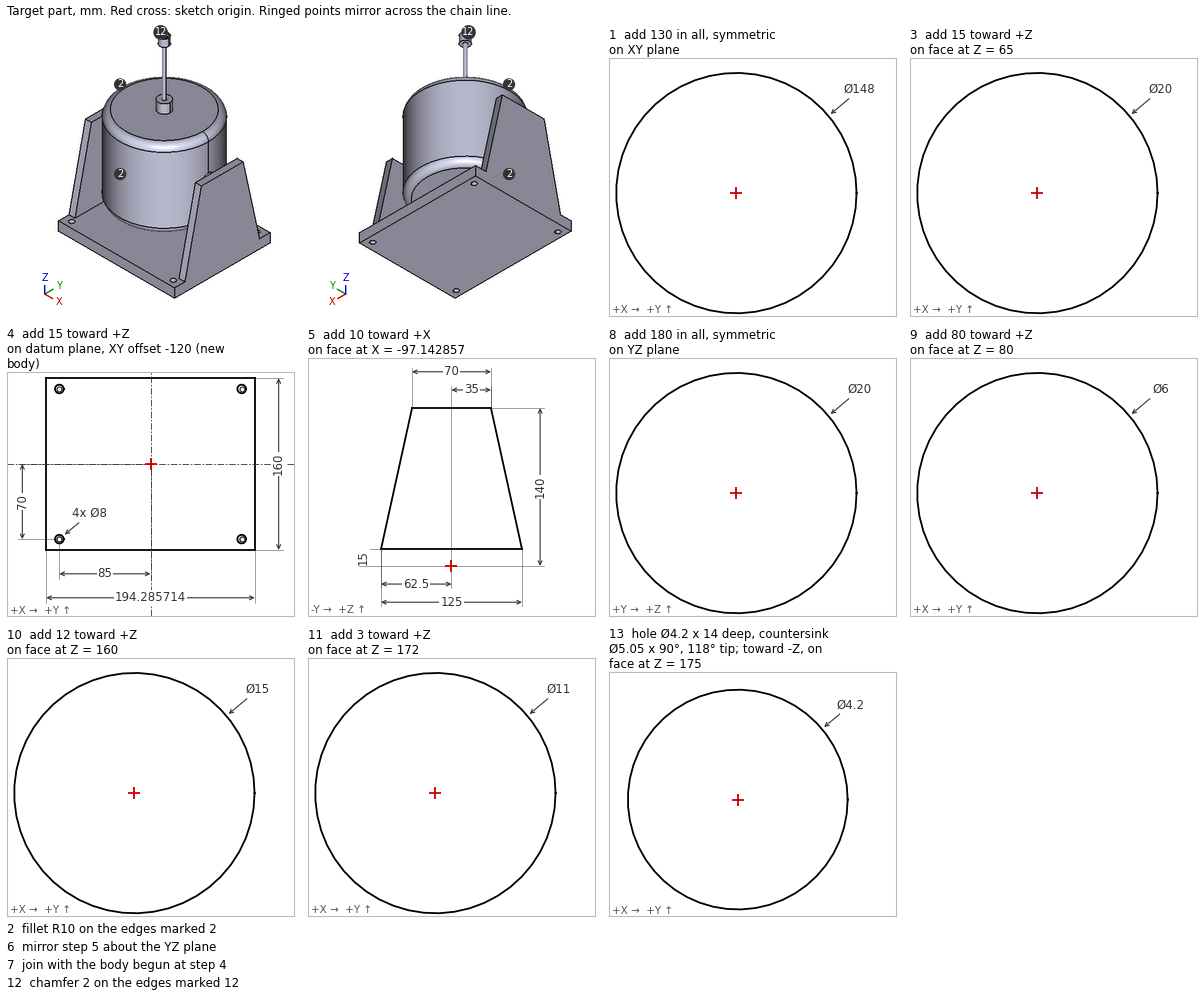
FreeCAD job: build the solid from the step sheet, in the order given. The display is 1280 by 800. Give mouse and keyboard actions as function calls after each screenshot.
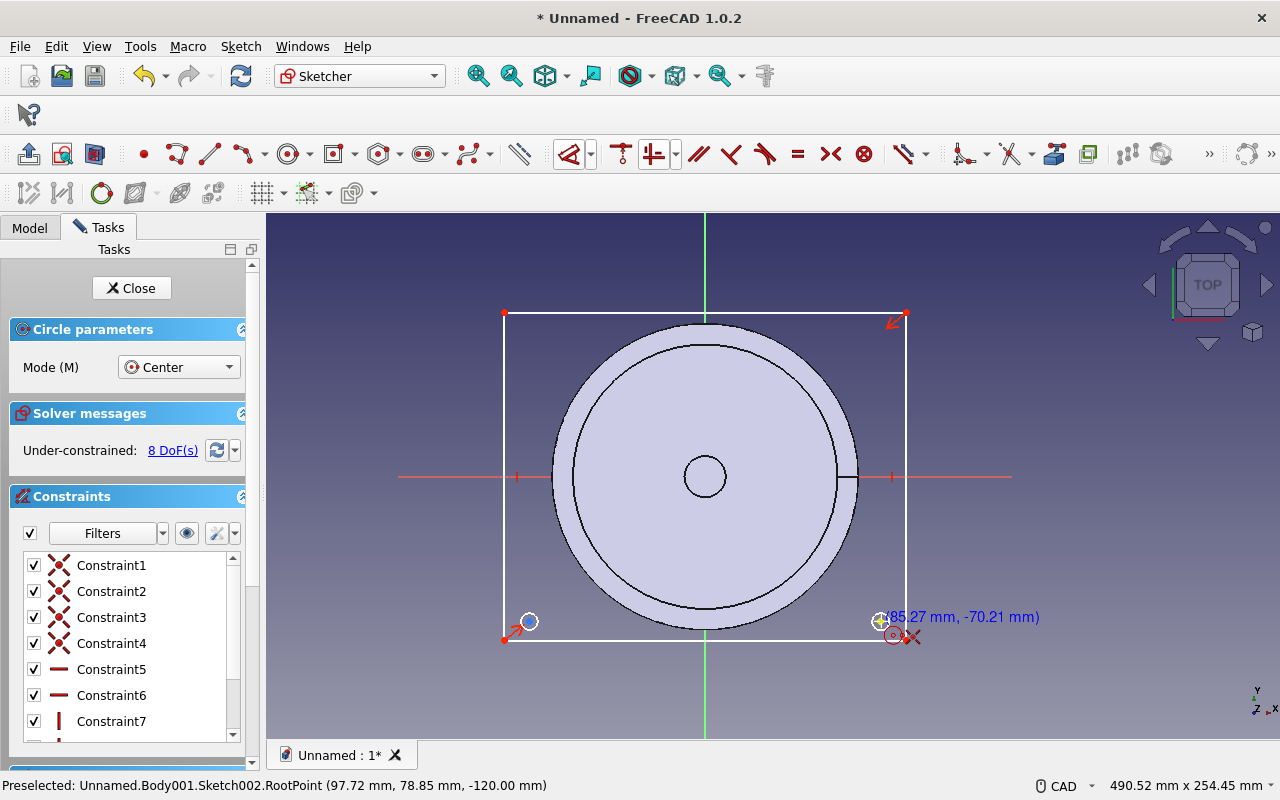
scroll(529, 332, up, 6)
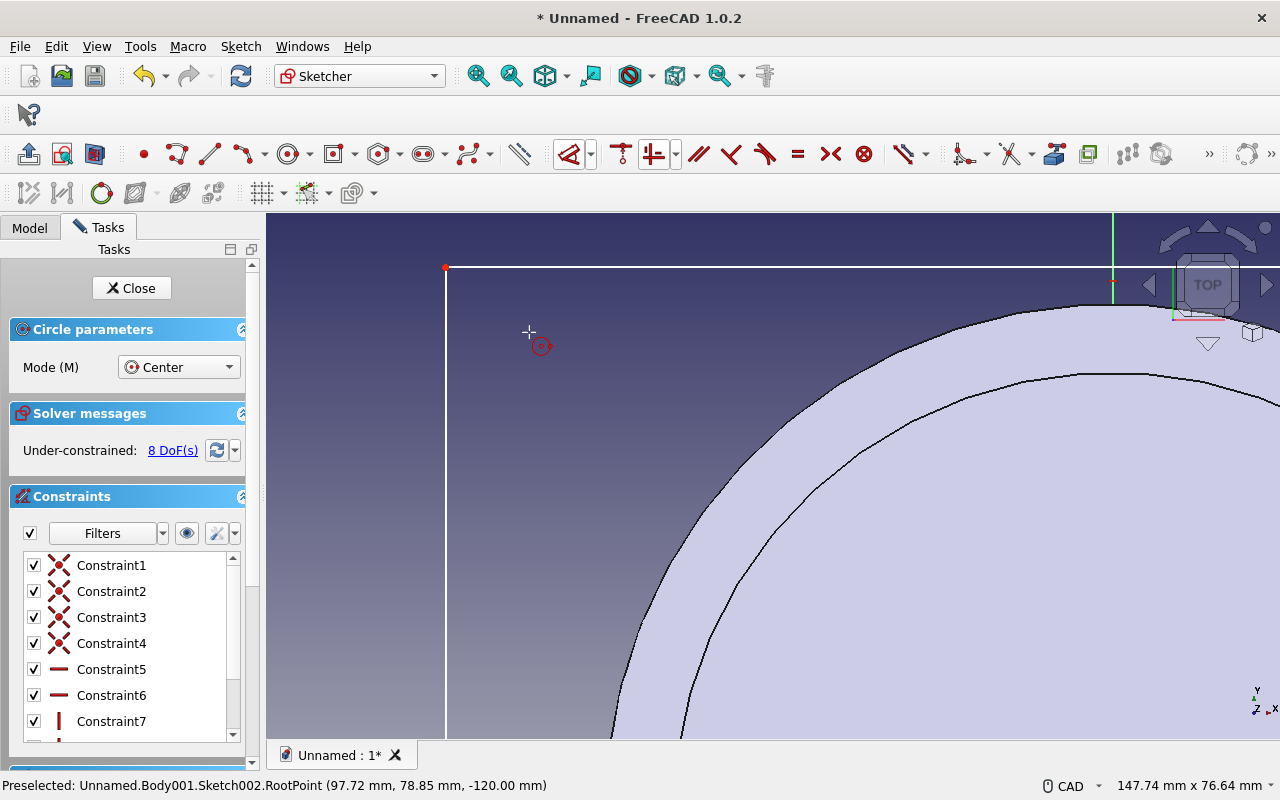
click(530, 331)
click(549, 312)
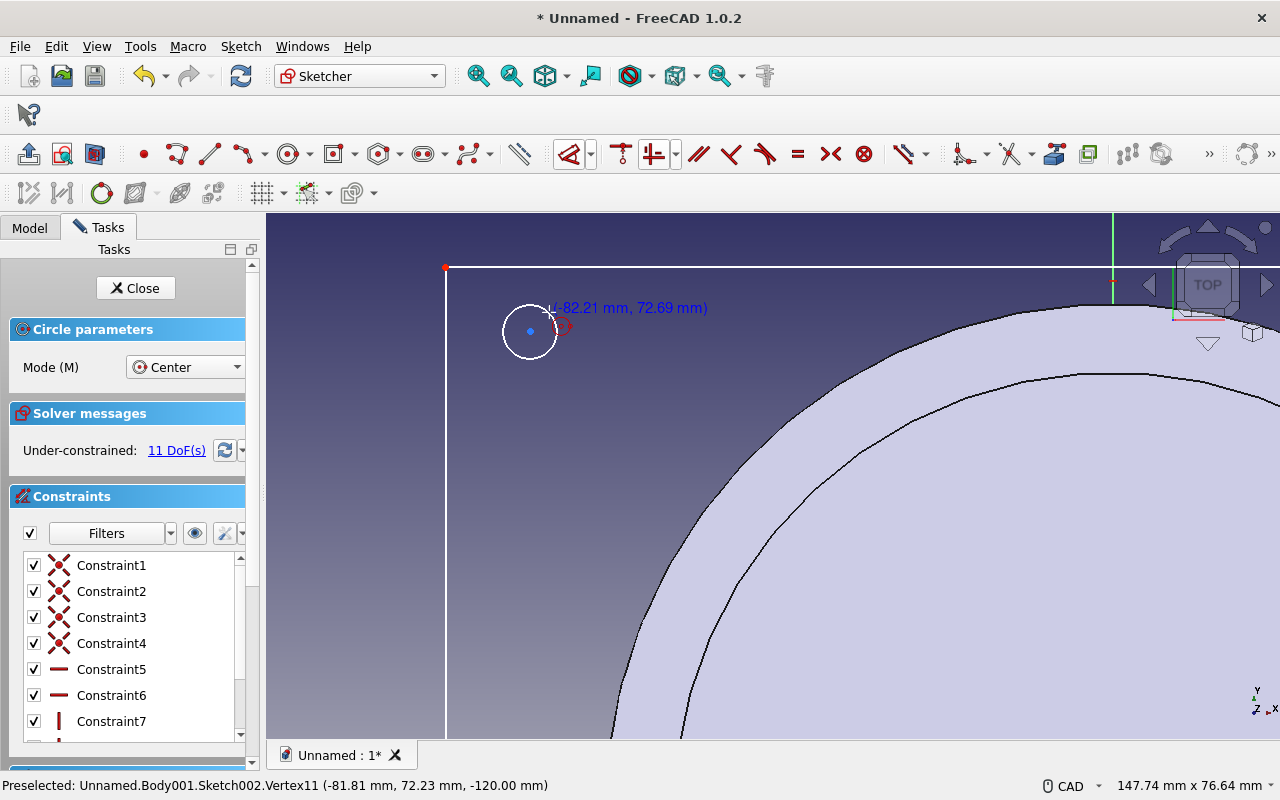
scroll(528, 331, down, 6)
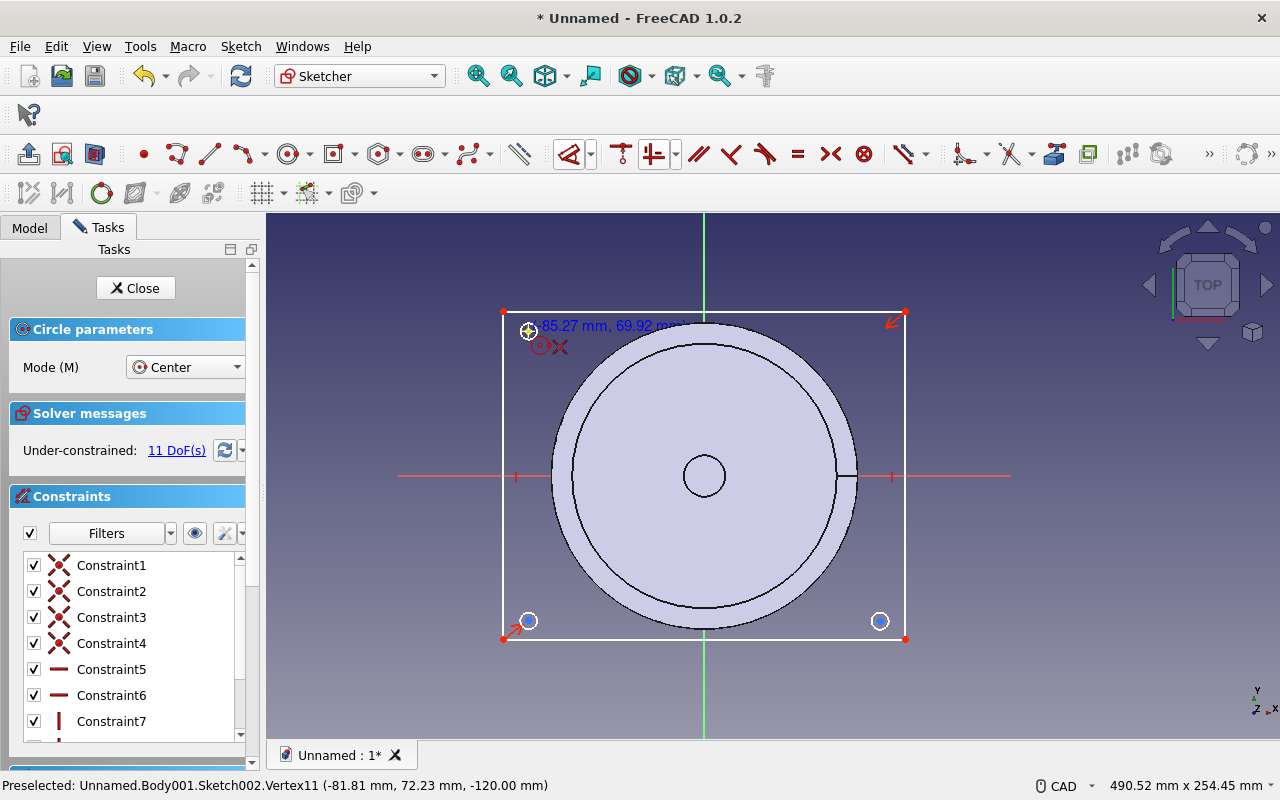
scroll(880, 331, up, 6)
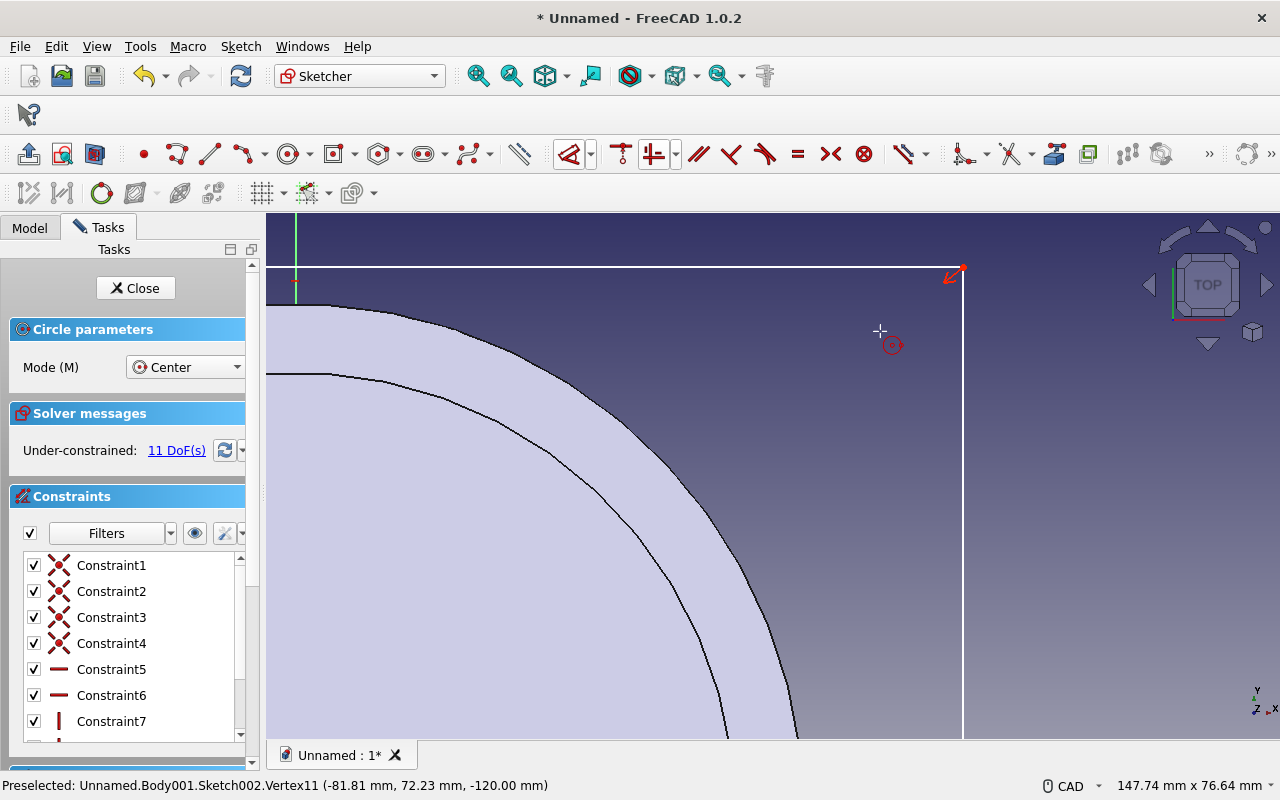
click(879, 331)
click(899, 312)
key(Escape)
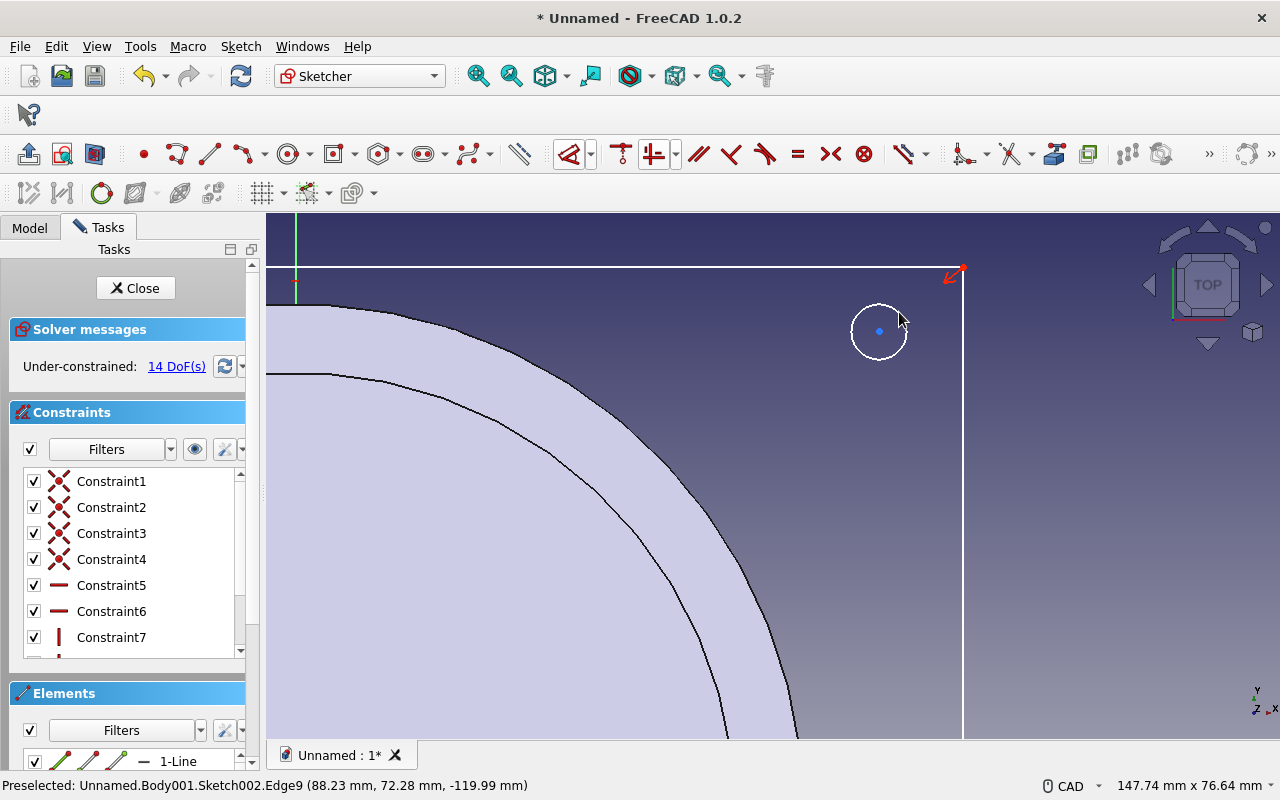
scroll(881, 331, down, 6)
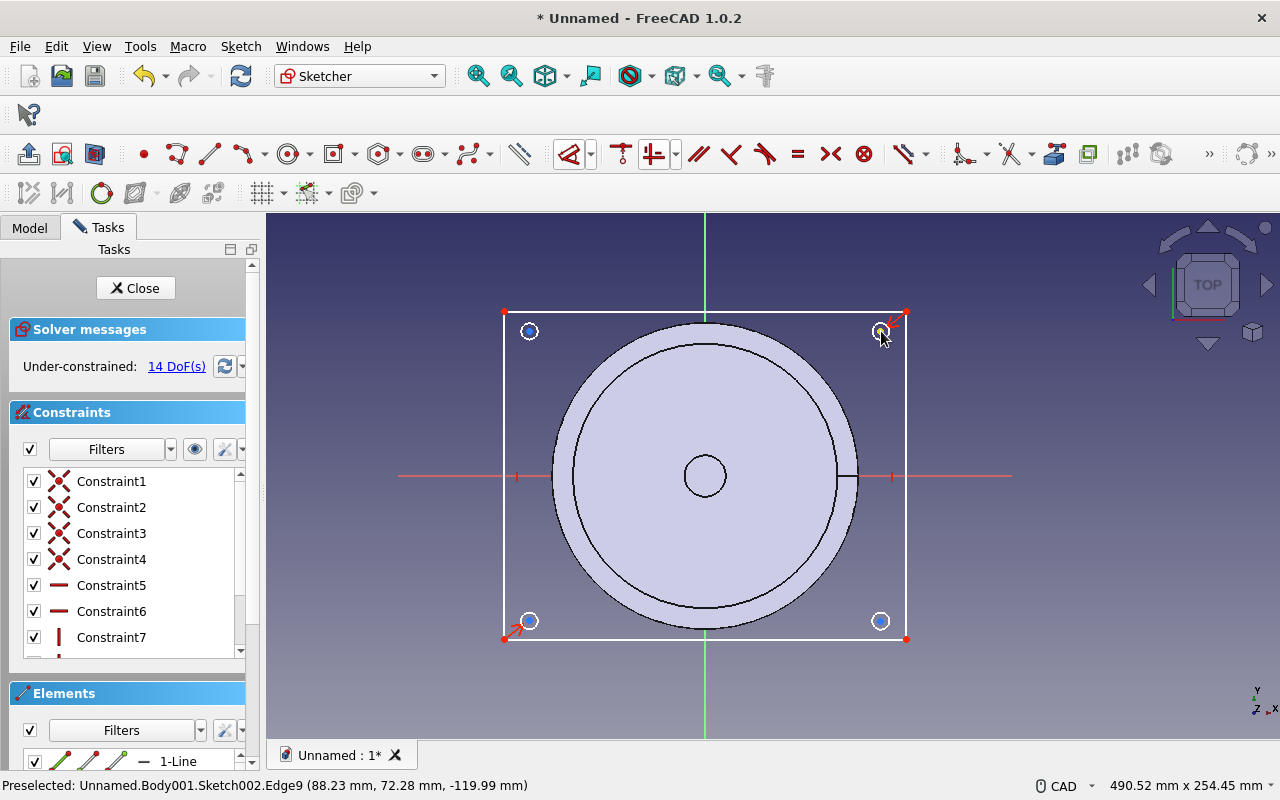
scroll(535, 615, up, 3)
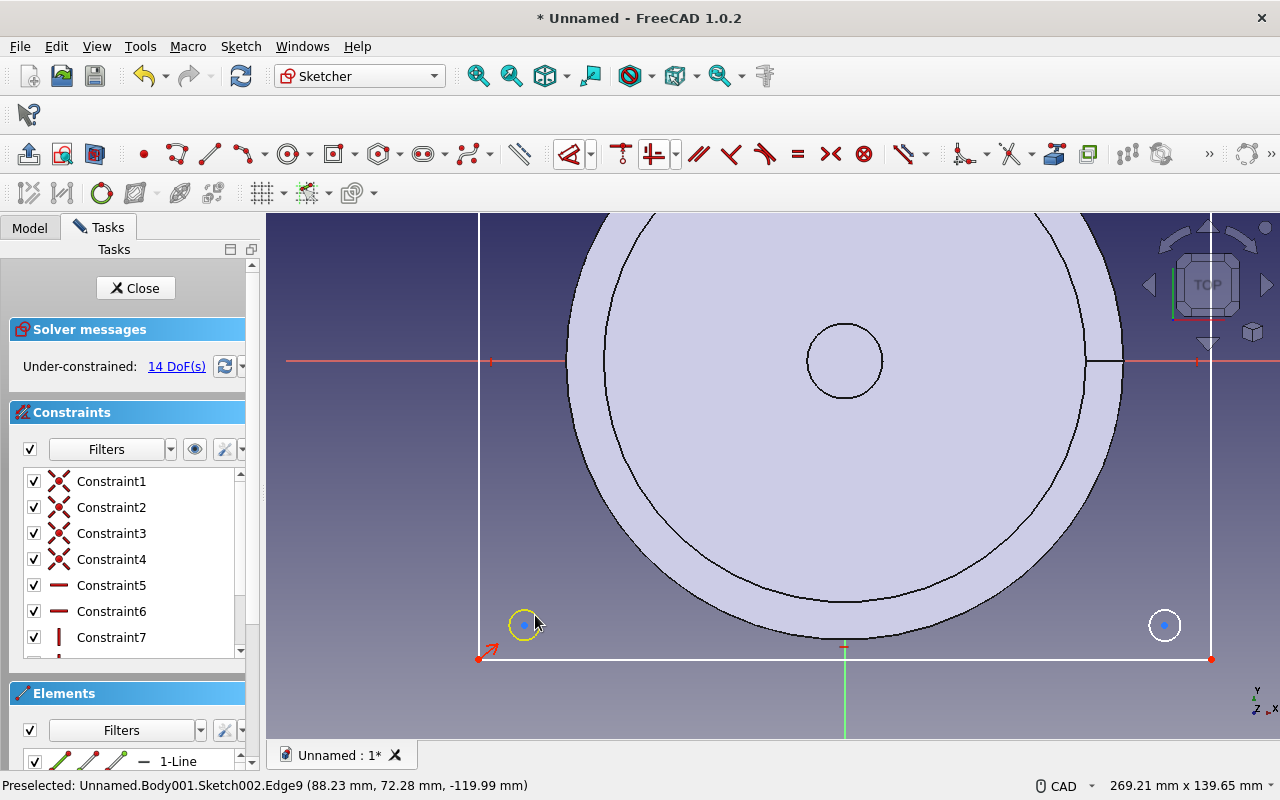
click(535, 614)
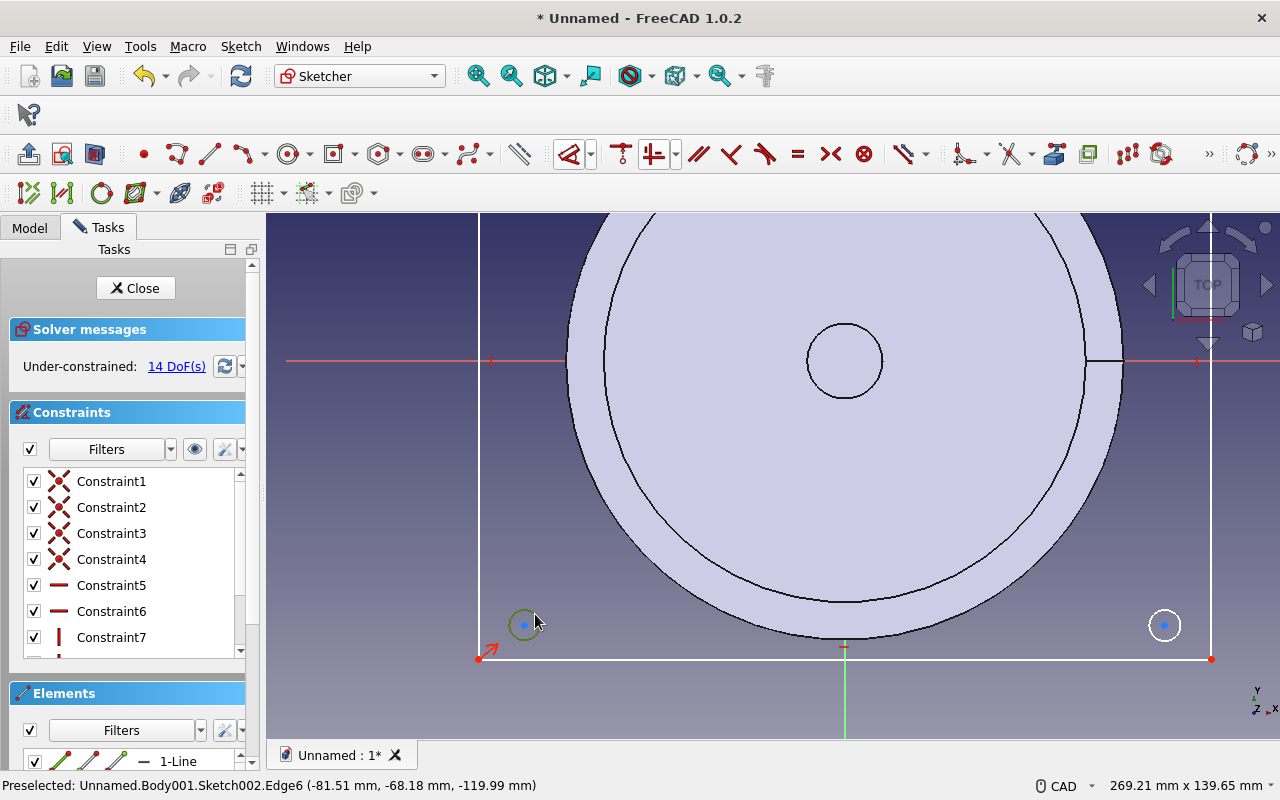
scroll(534, 616, down, 3)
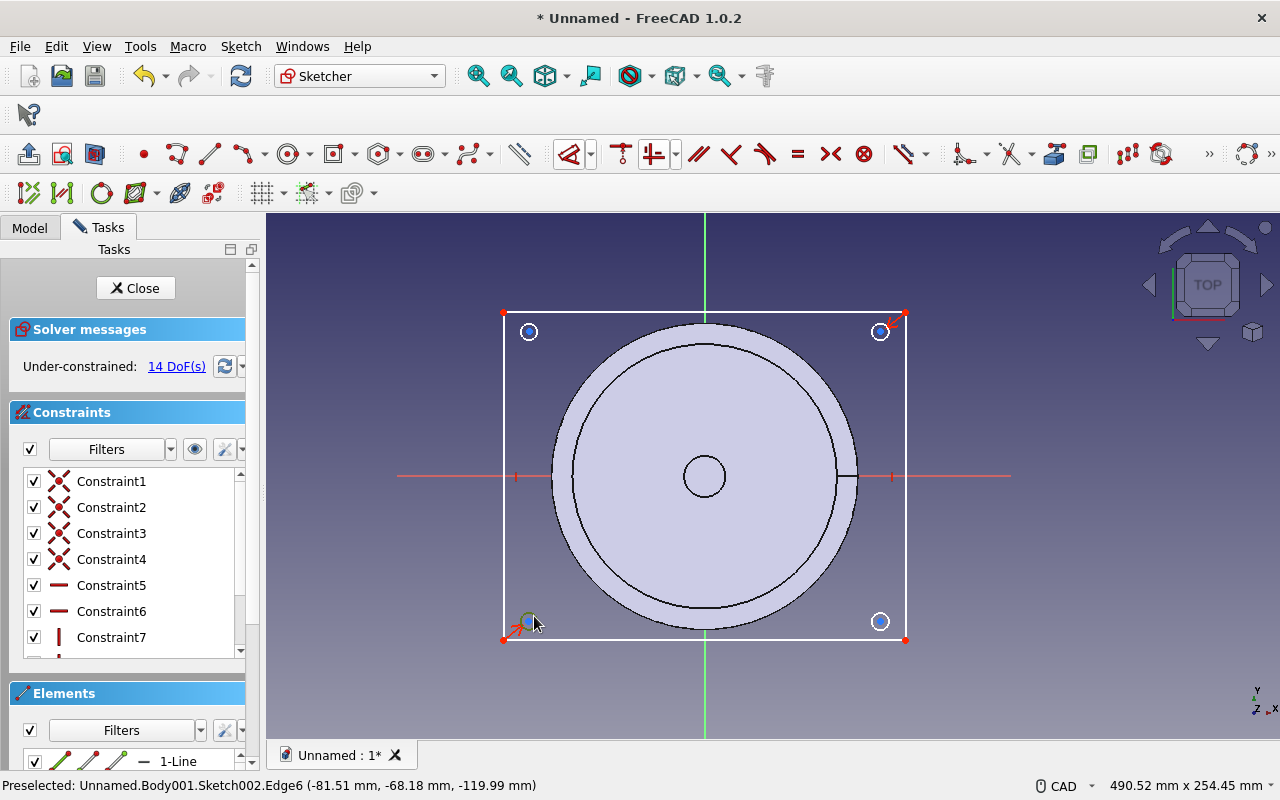
scroll(886, 616, up, 3)